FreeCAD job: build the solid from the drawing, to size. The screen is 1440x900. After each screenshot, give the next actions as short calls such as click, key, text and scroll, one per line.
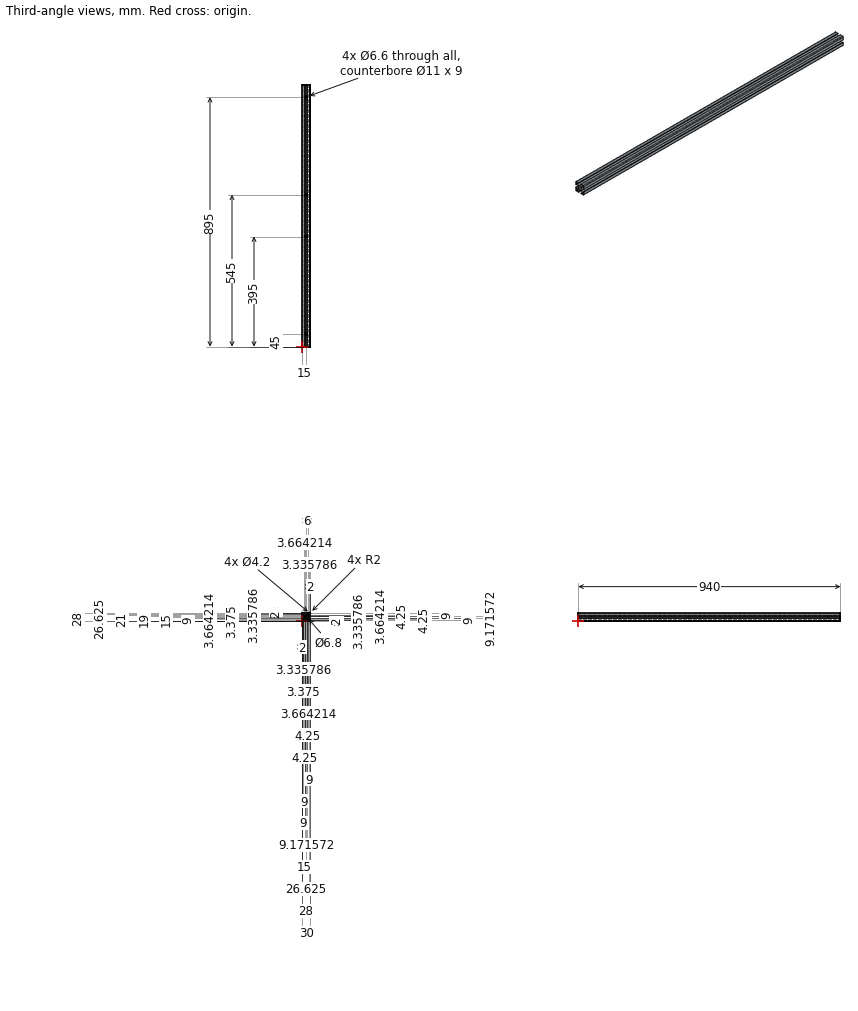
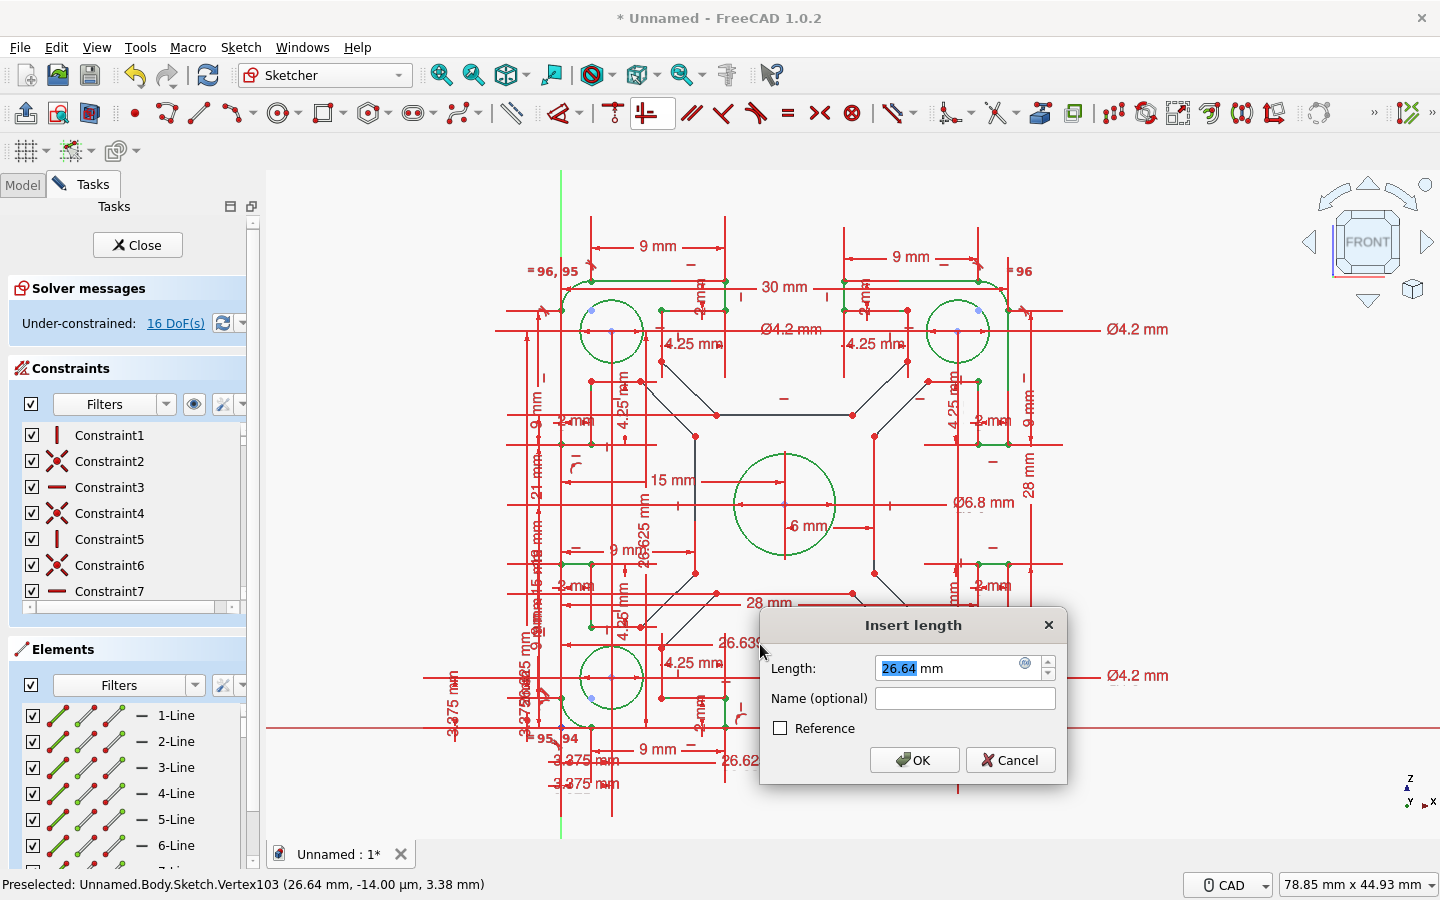
text(26.625)
key(Return)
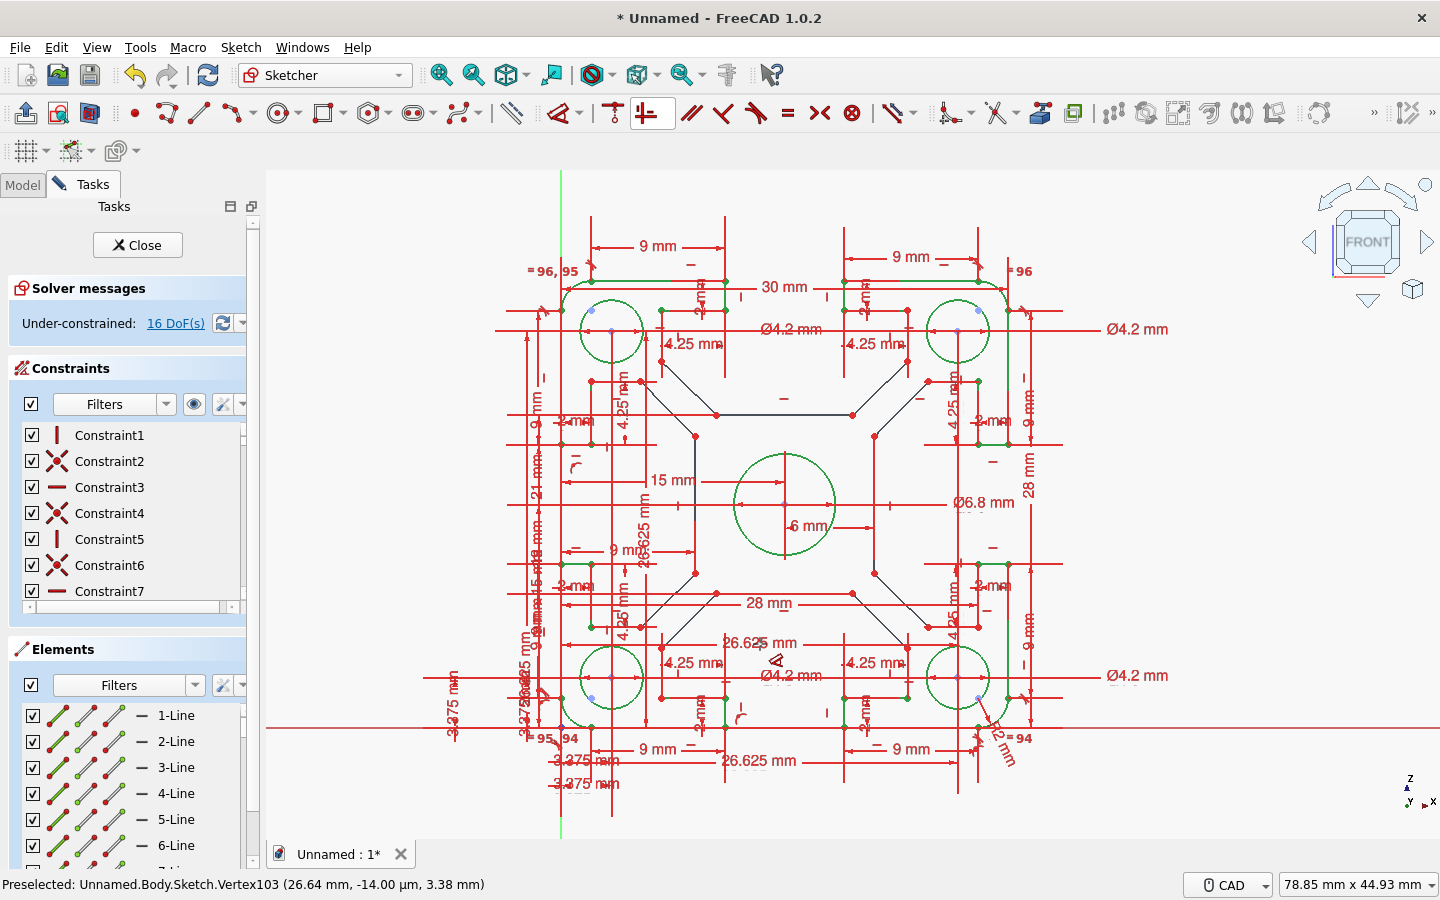
click(963, 382)
click(954, 348)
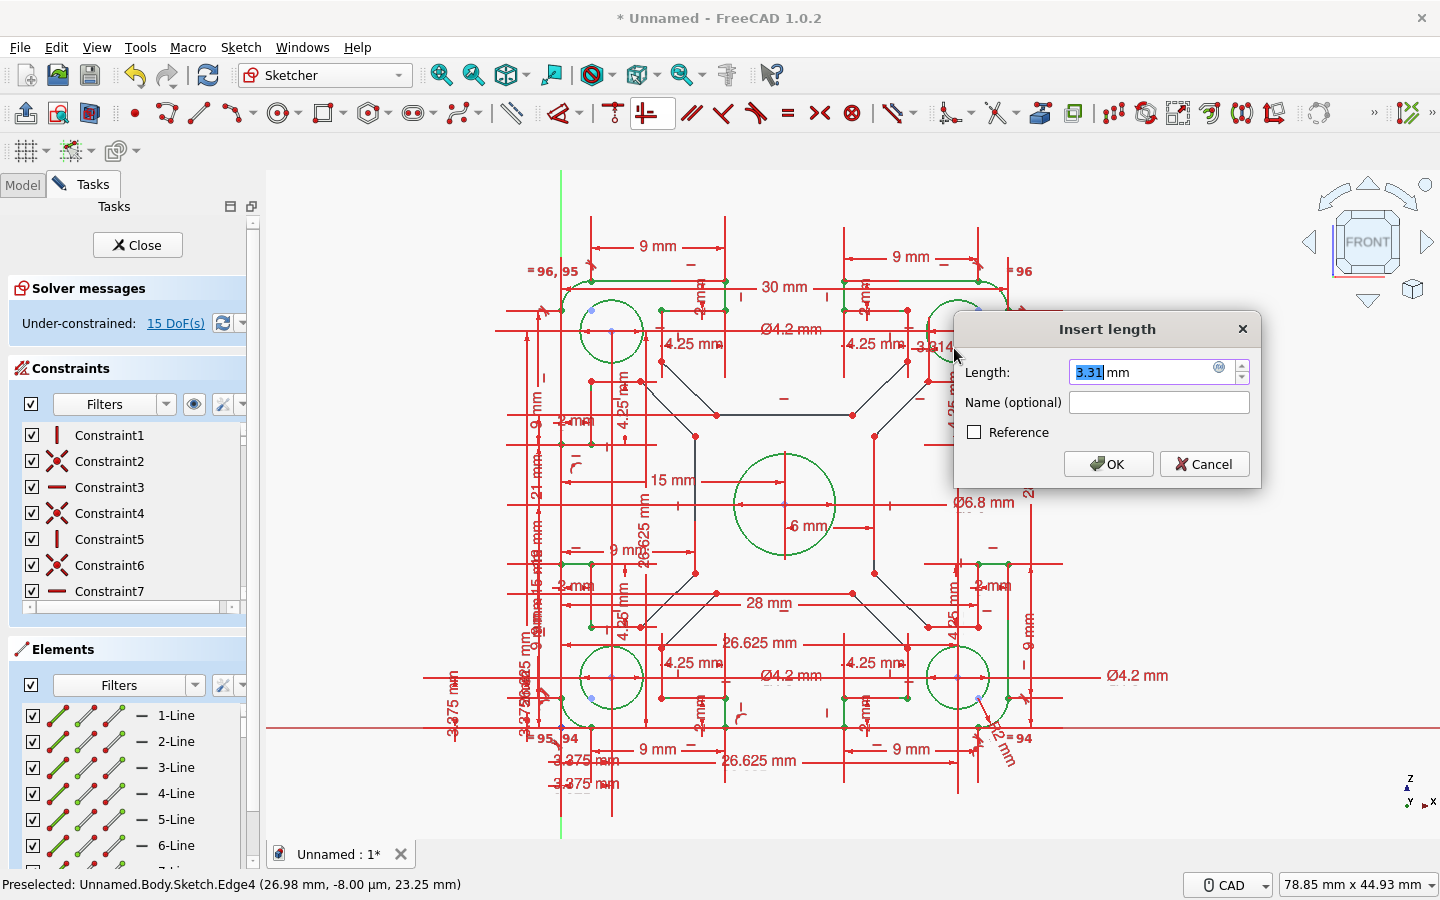
text(3.335786)
key(Return)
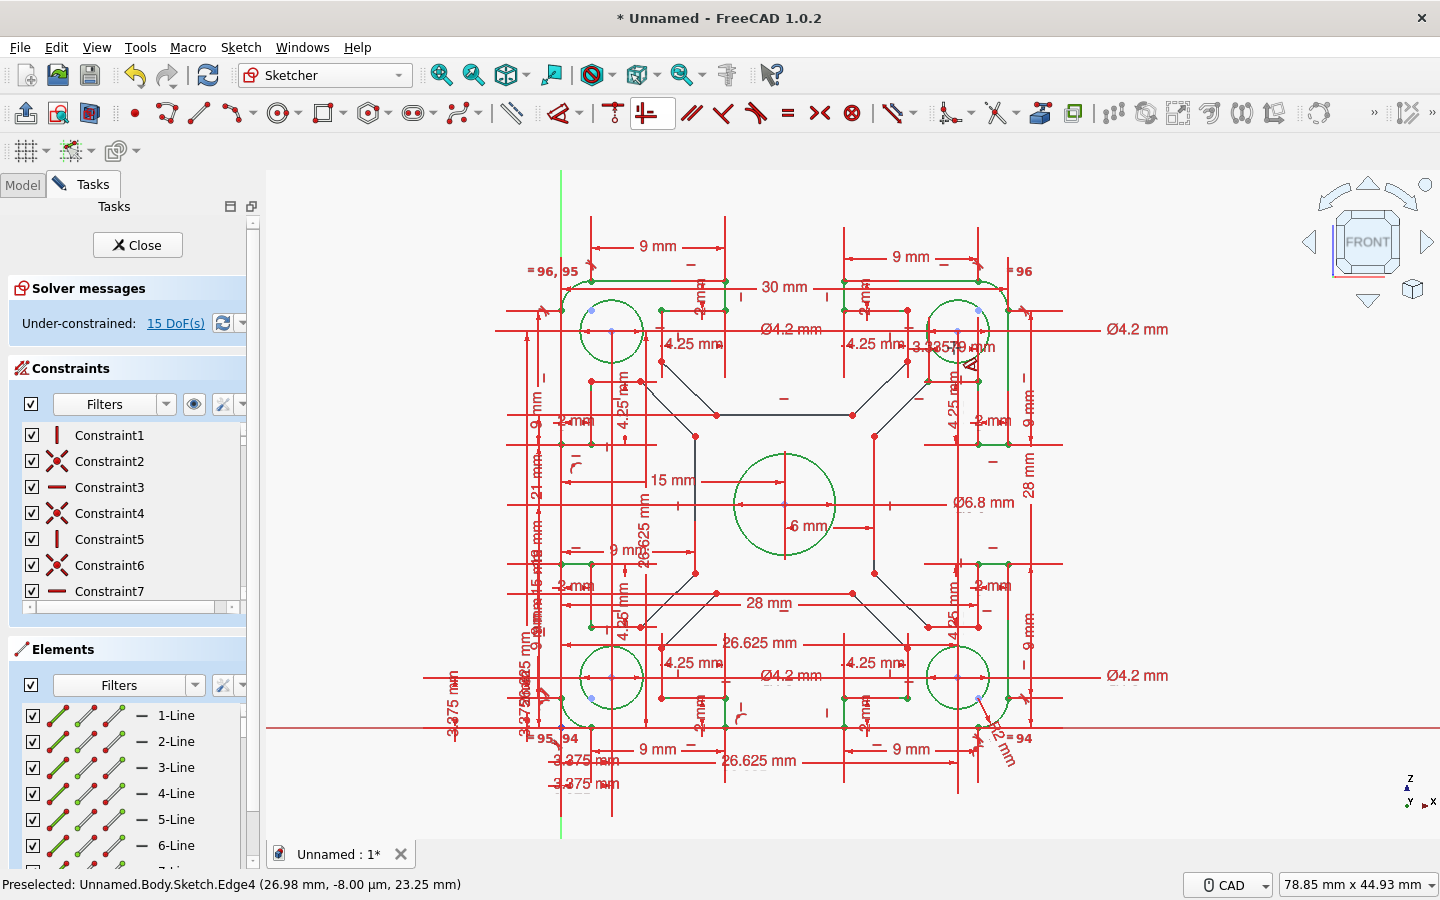
click(874, 478)
click(908, 505)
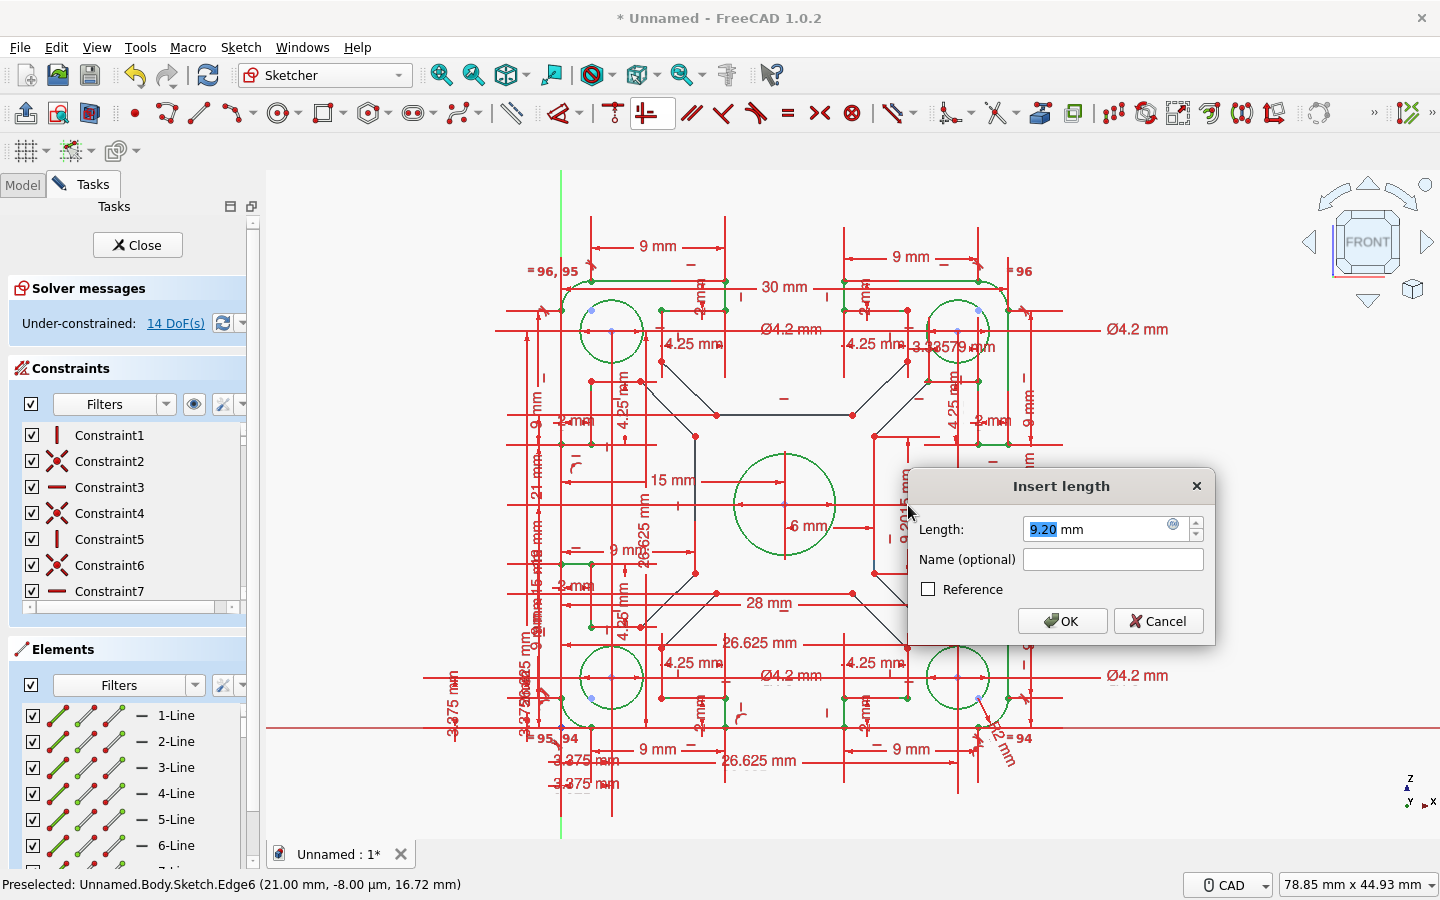
text(9.171572)
key(Return)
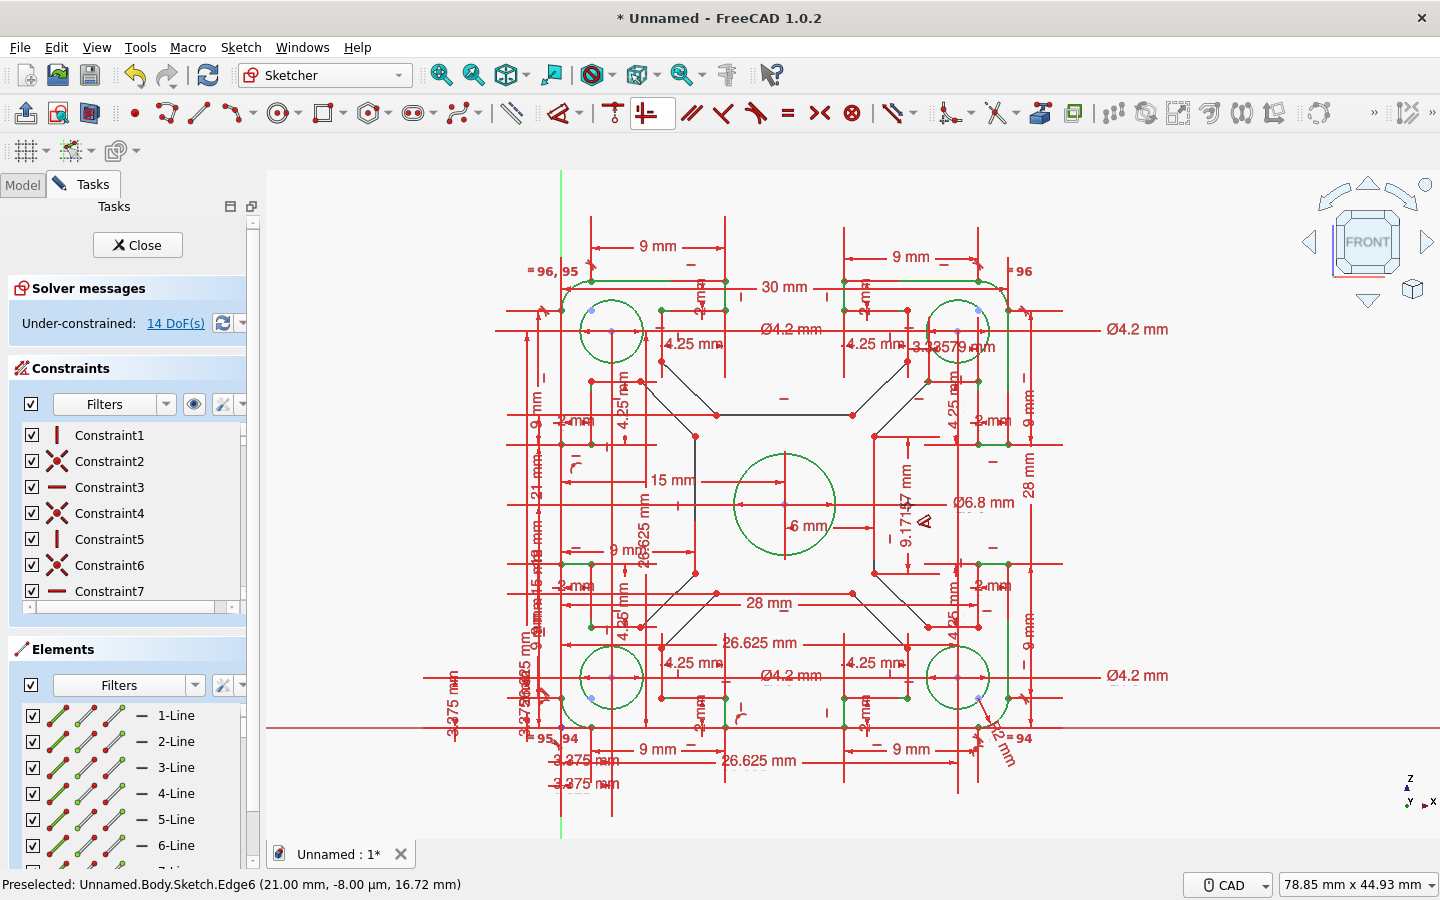
click(944, 627)
click(954, 661)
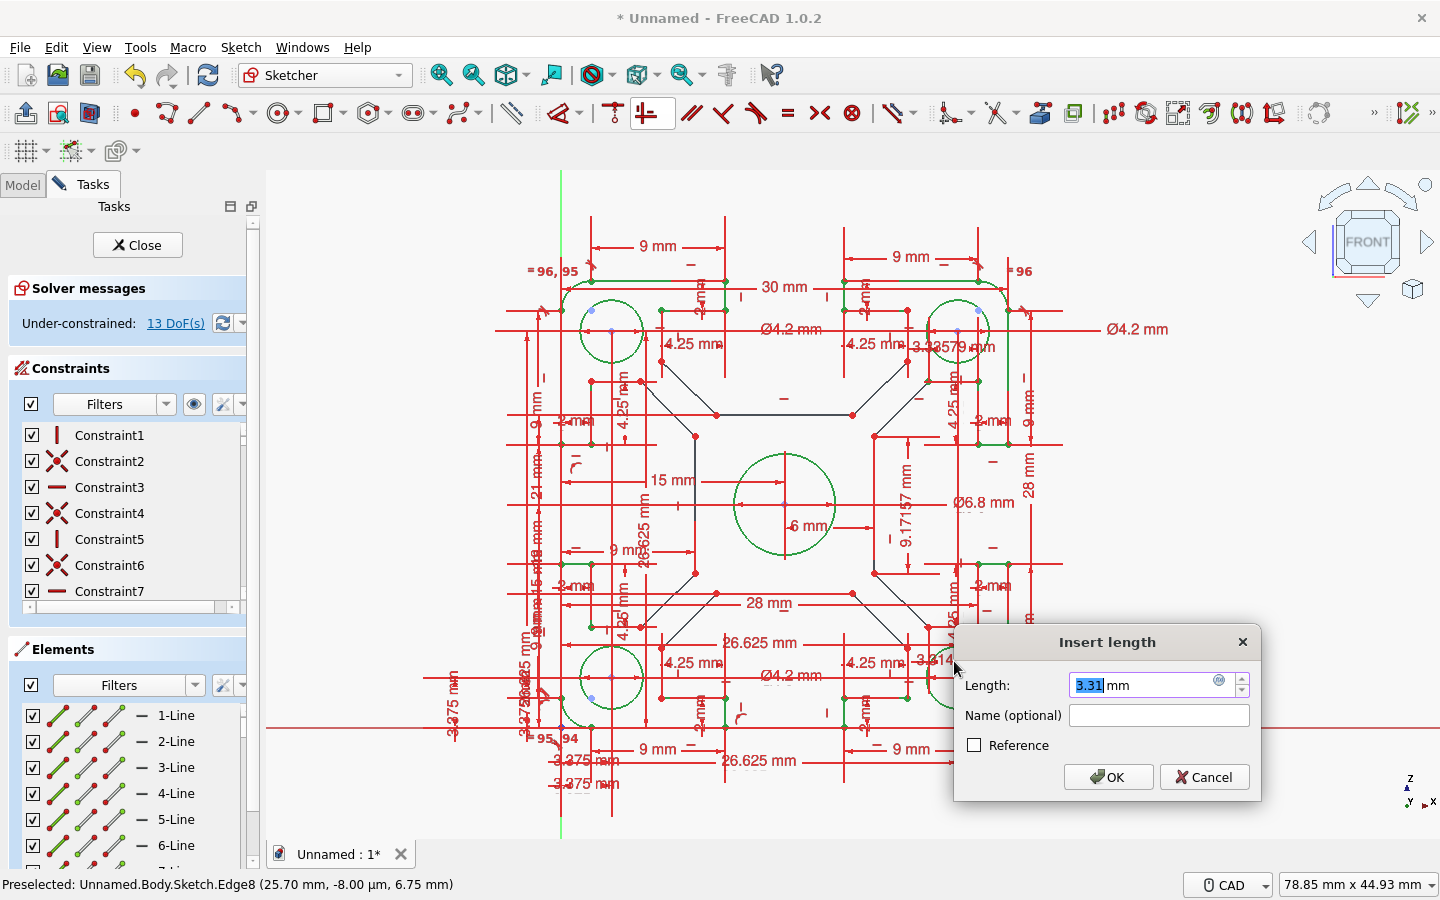
text(3.335786)
key(Return)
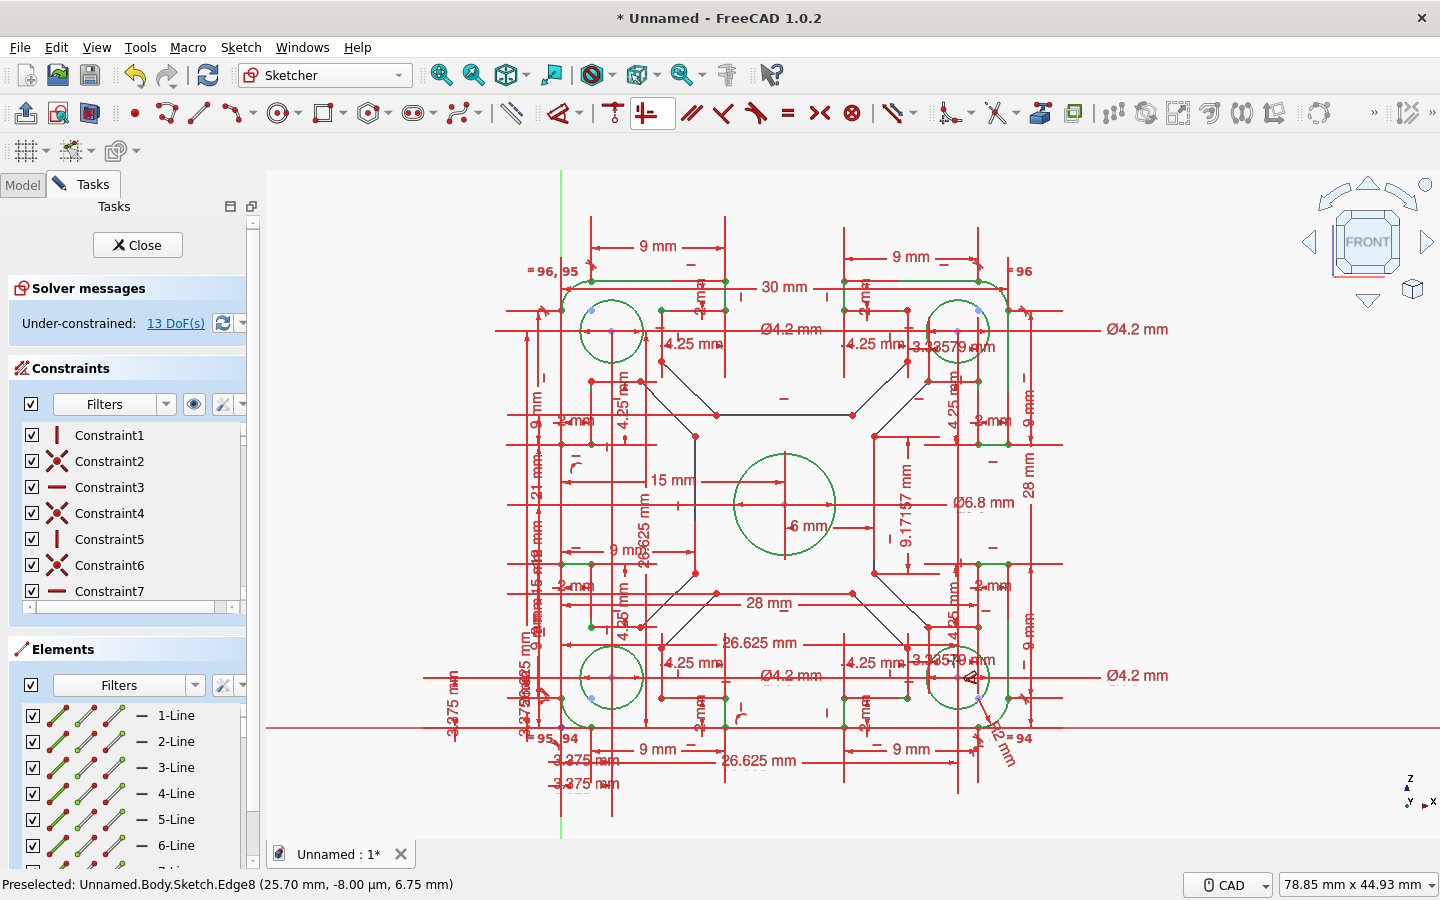
click(908, 683)
click(942, 685)